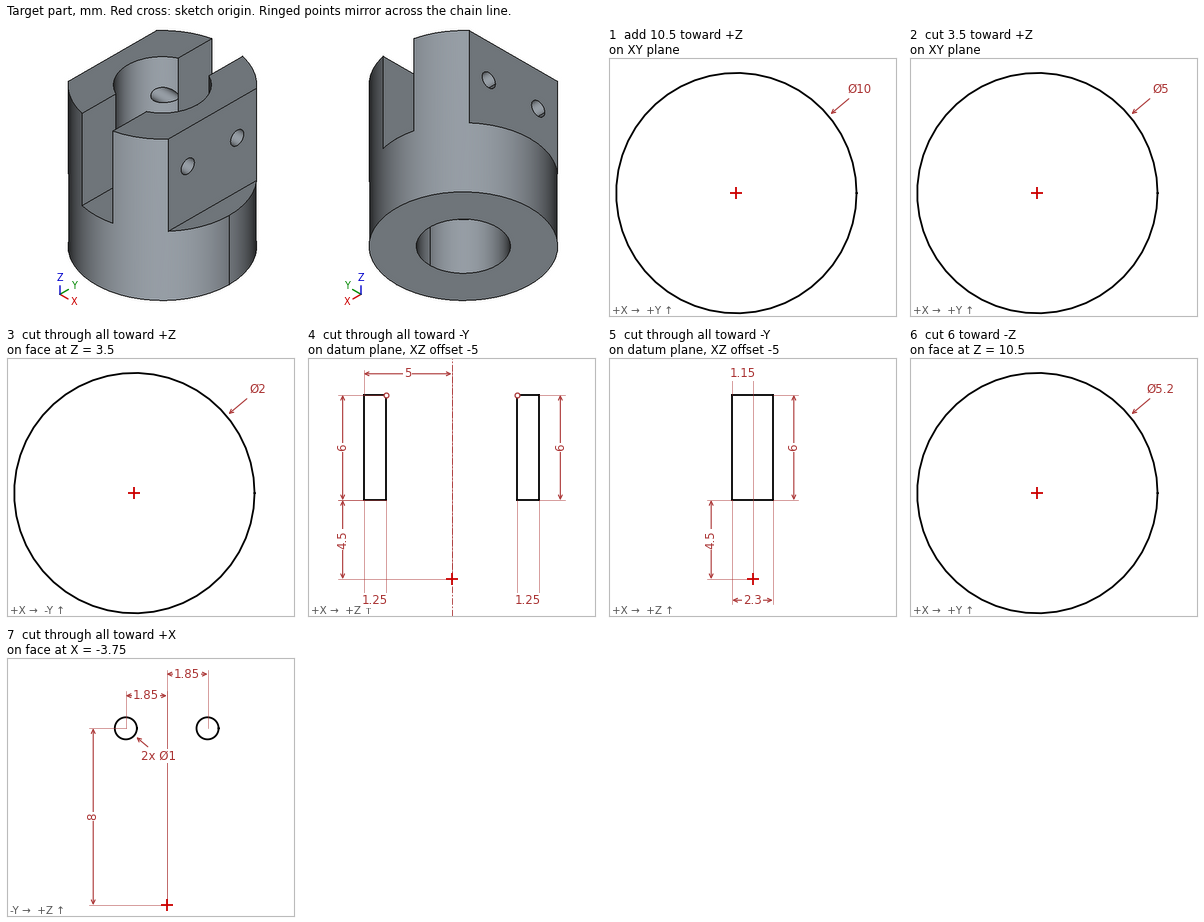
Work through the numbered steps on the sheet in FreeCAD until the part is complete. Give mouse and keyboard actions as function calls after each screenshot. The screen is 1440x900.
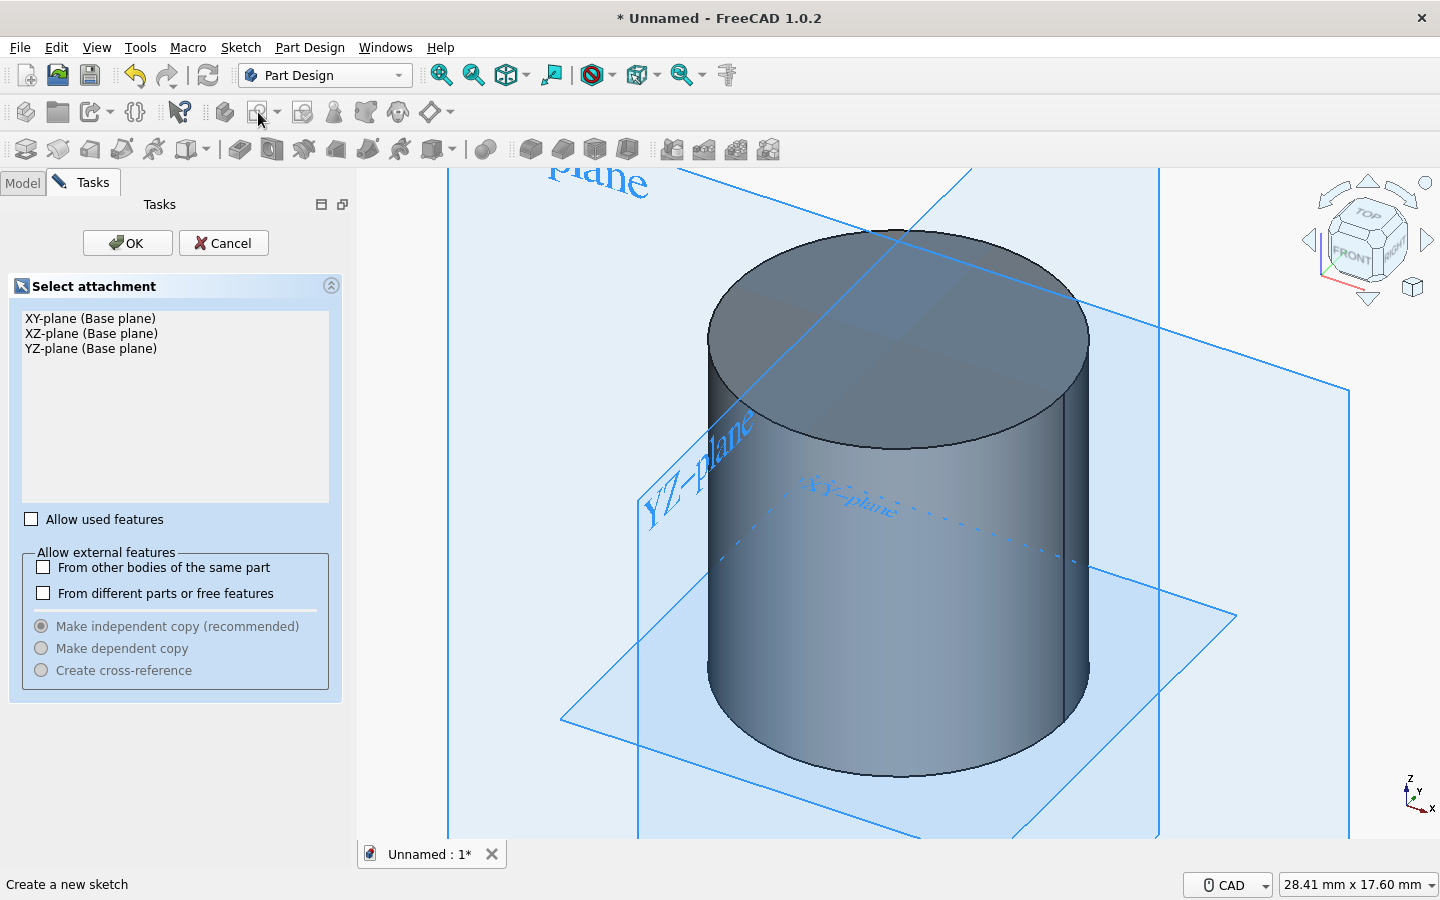
click(82, 318)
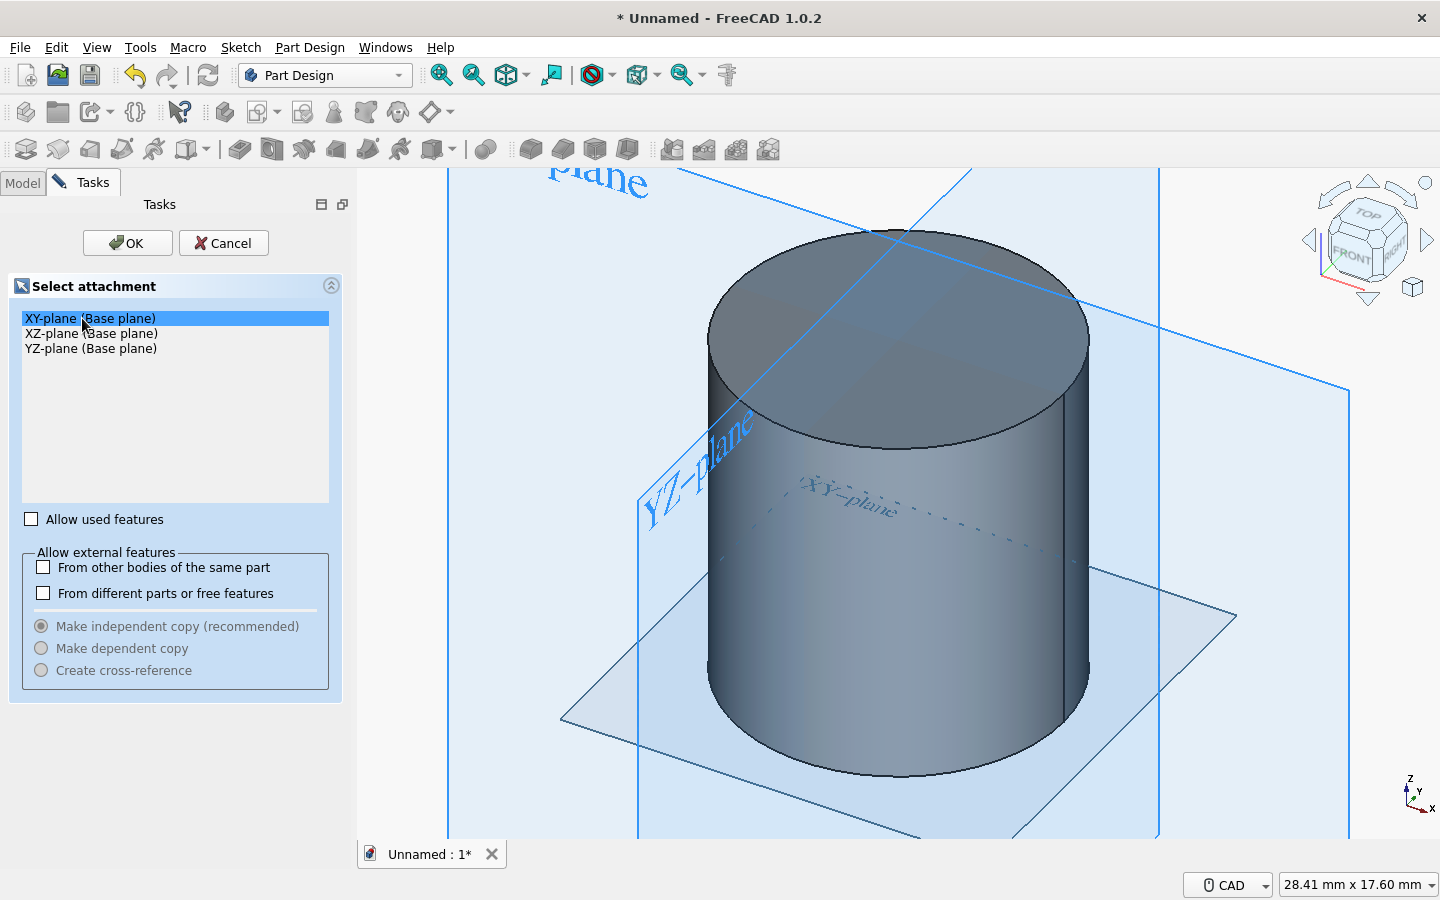
click(128, 243)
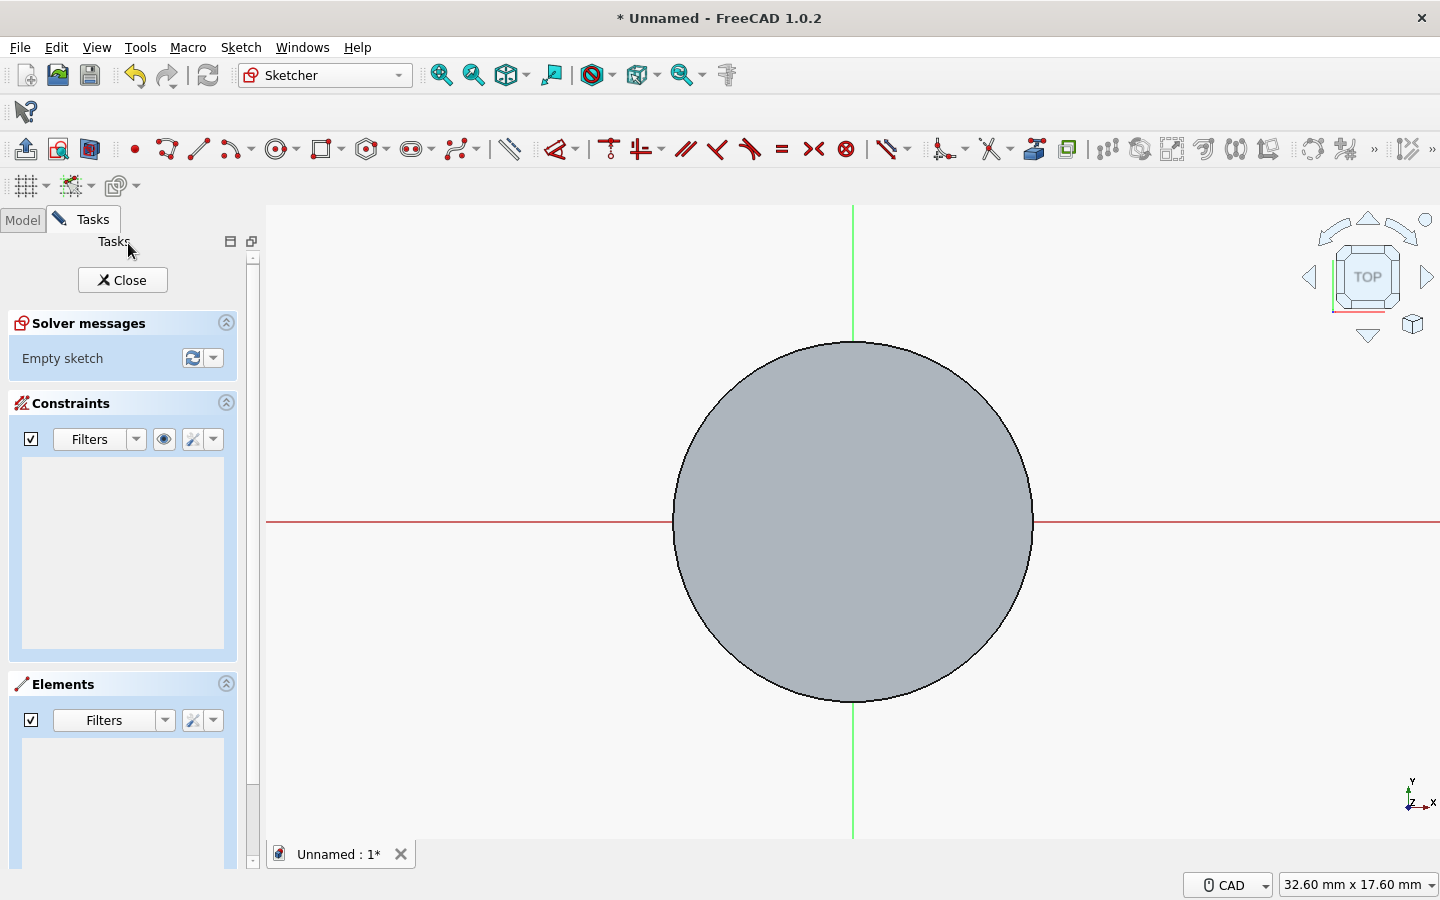
key(q)
key(s)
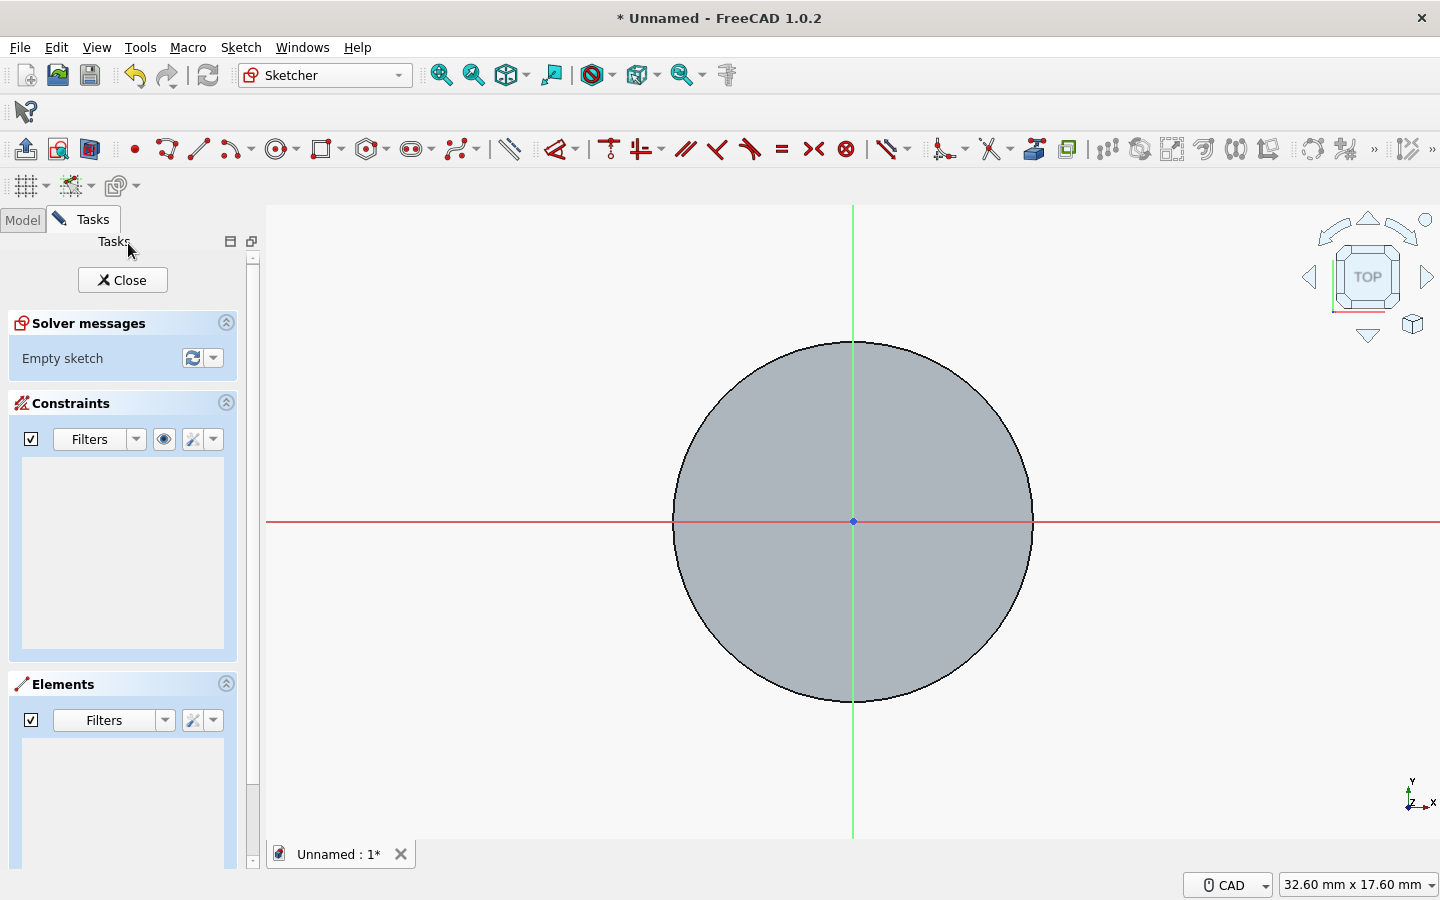
scroll(909, 522, up, 4)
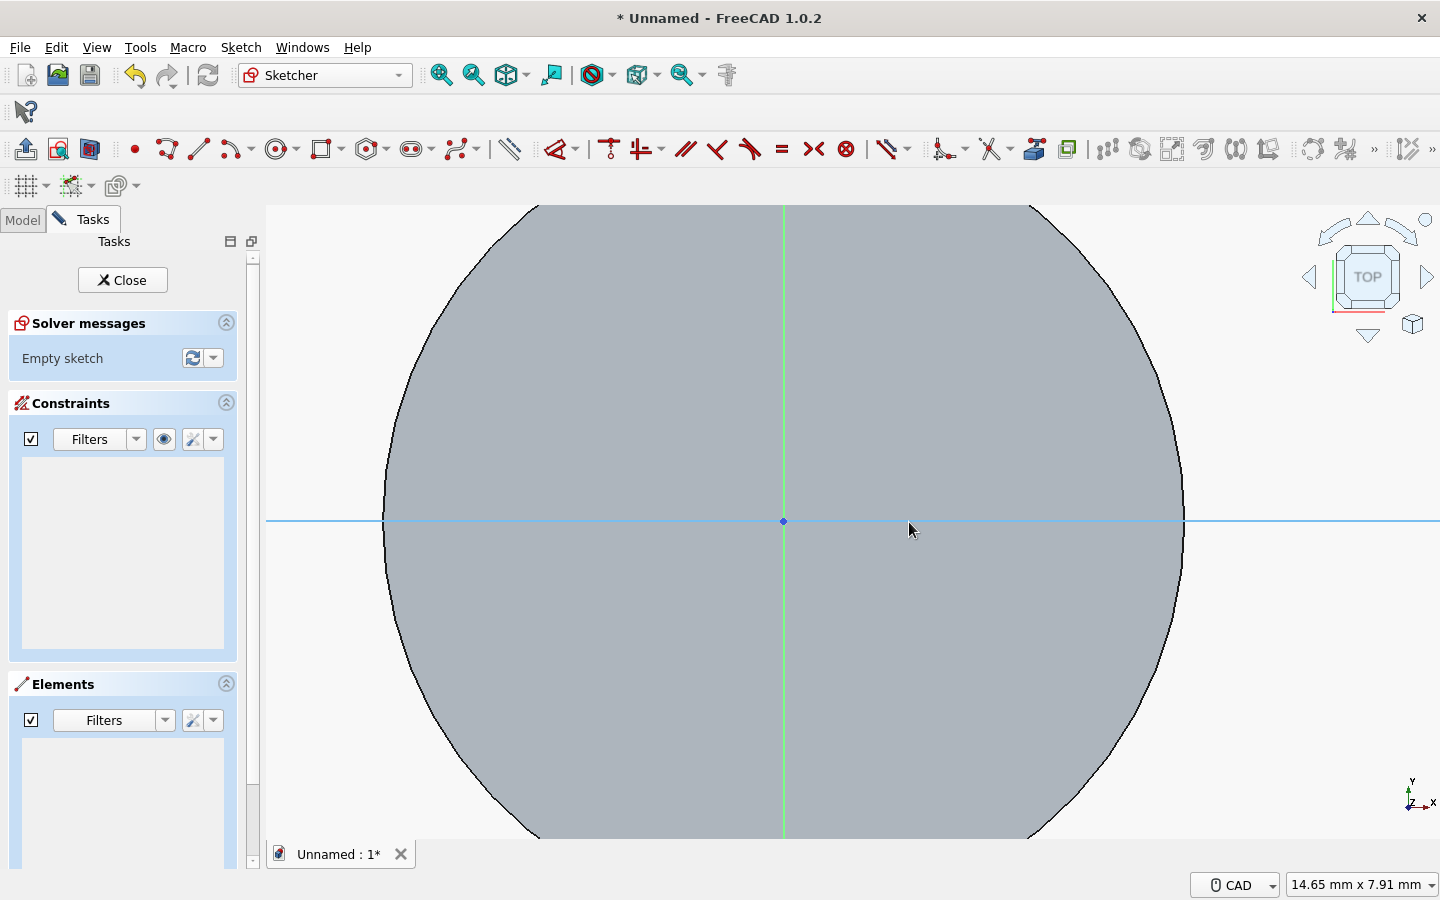
click(276, 150)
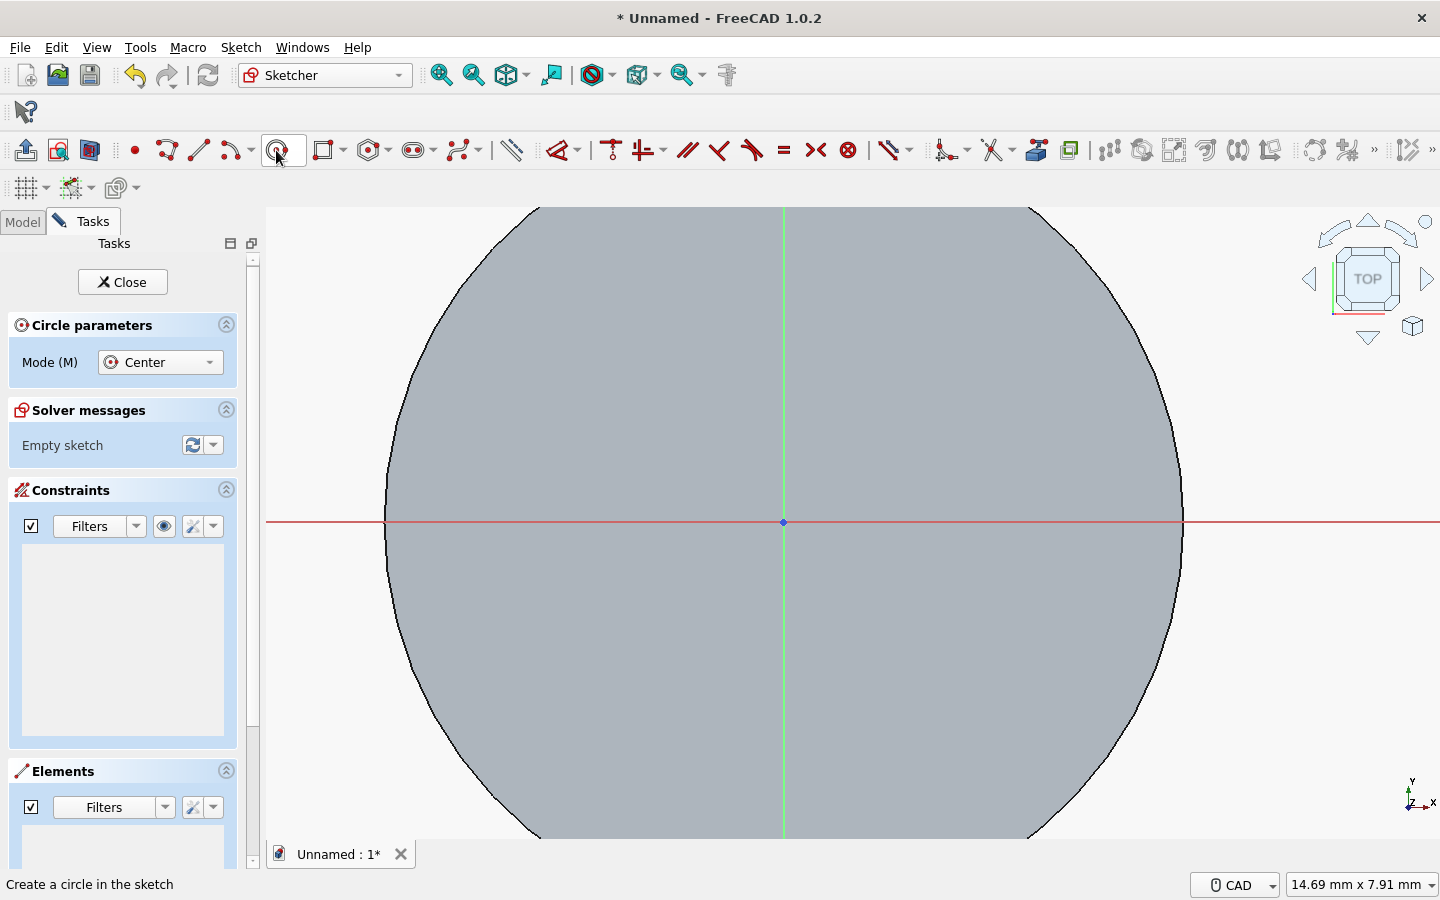
click(784, 522)
move(925, 381)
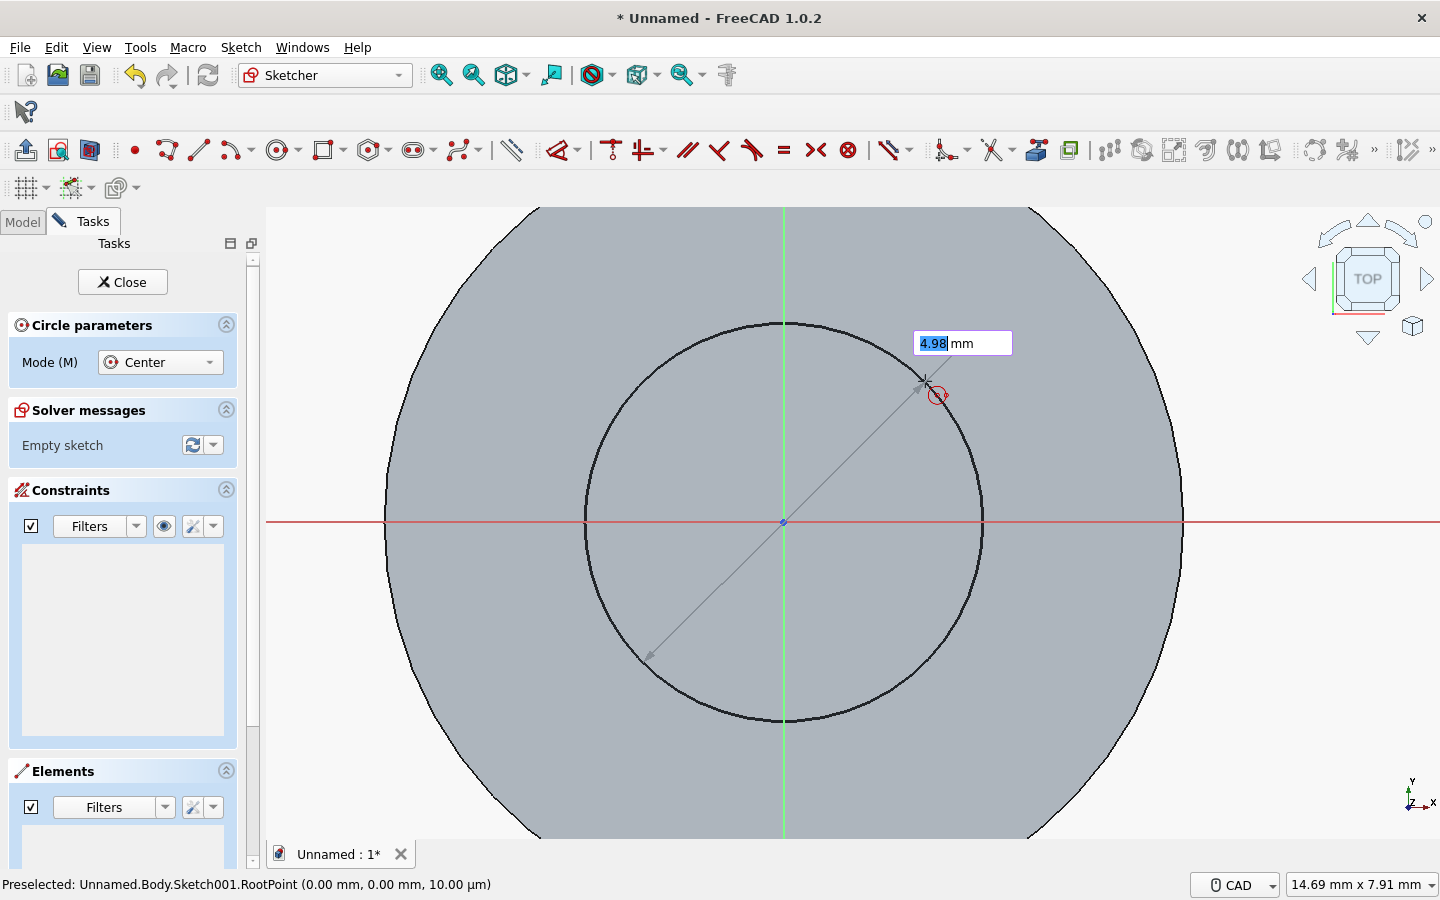
text(5)
key(Return)
key(Escape)